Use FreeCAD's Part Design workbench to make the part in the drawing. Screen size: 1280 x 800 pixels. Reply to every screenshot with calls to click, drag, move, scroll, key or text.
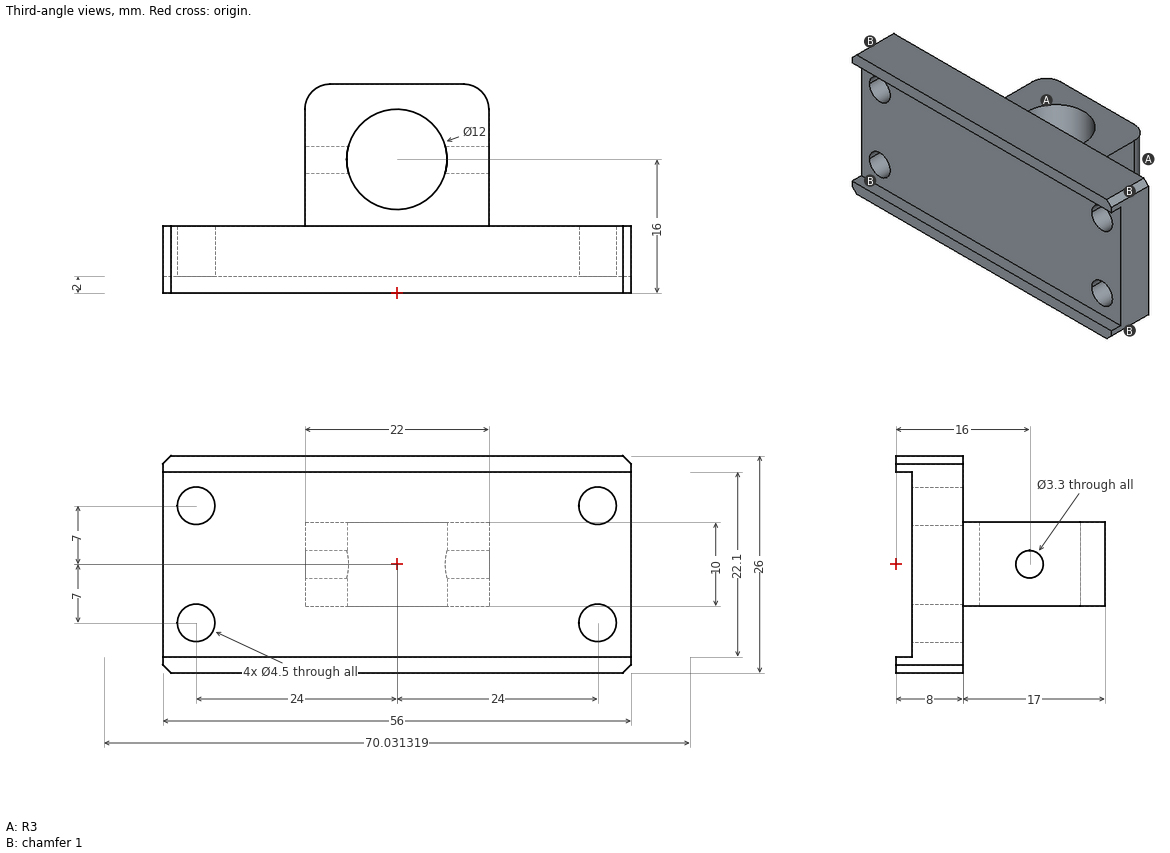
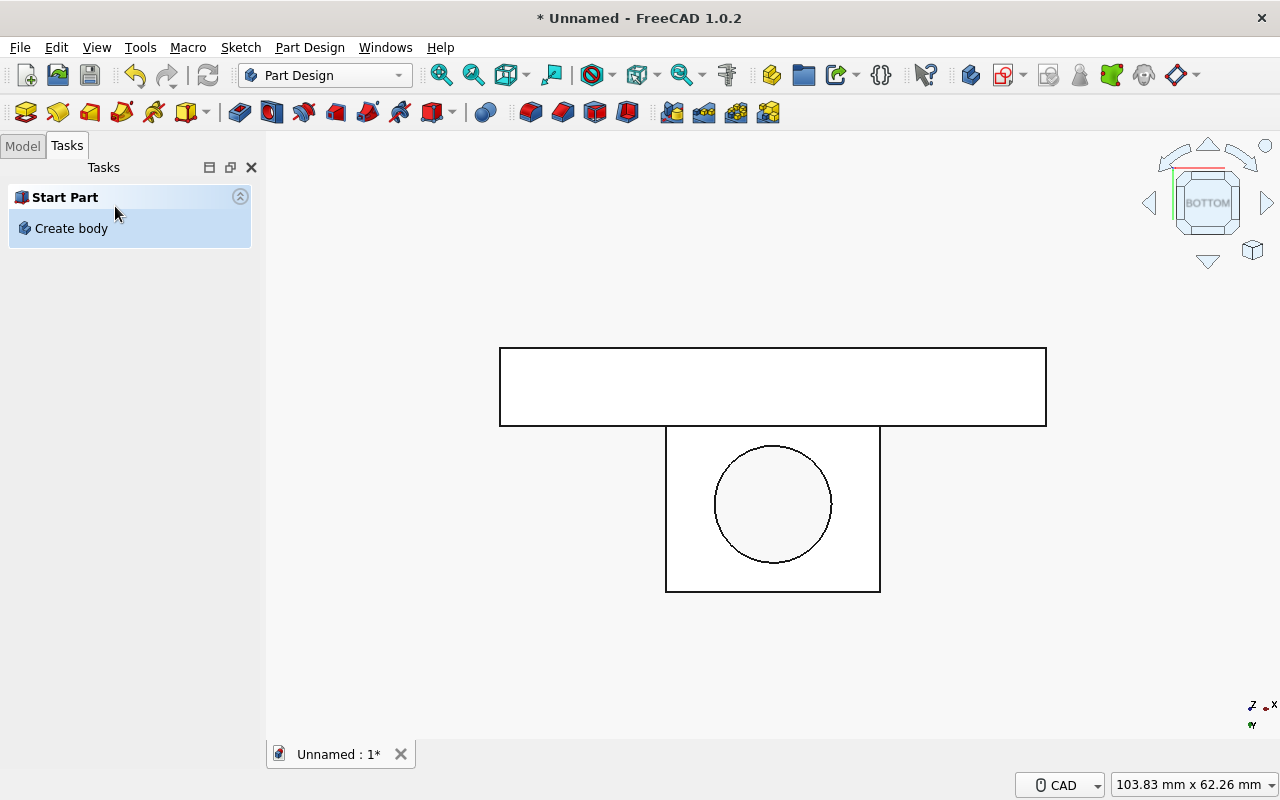
key(4)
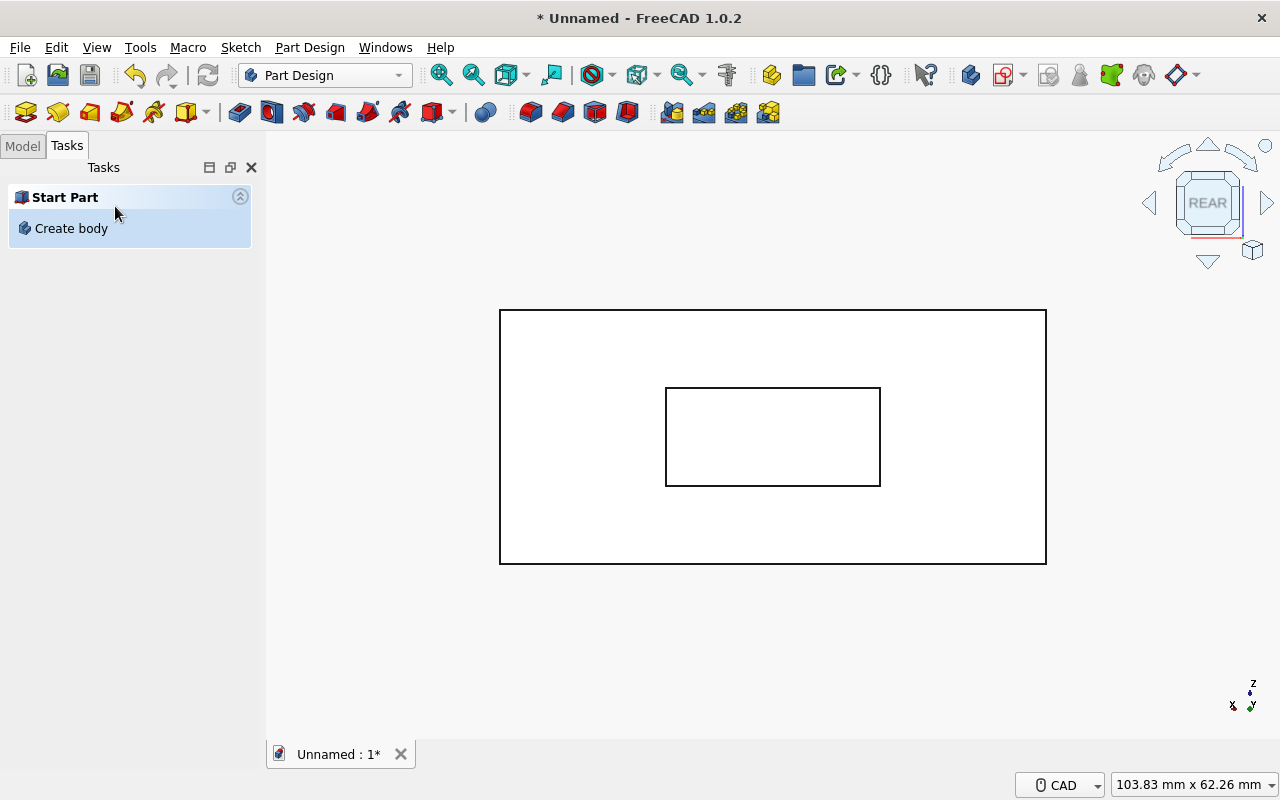
click(617, 508)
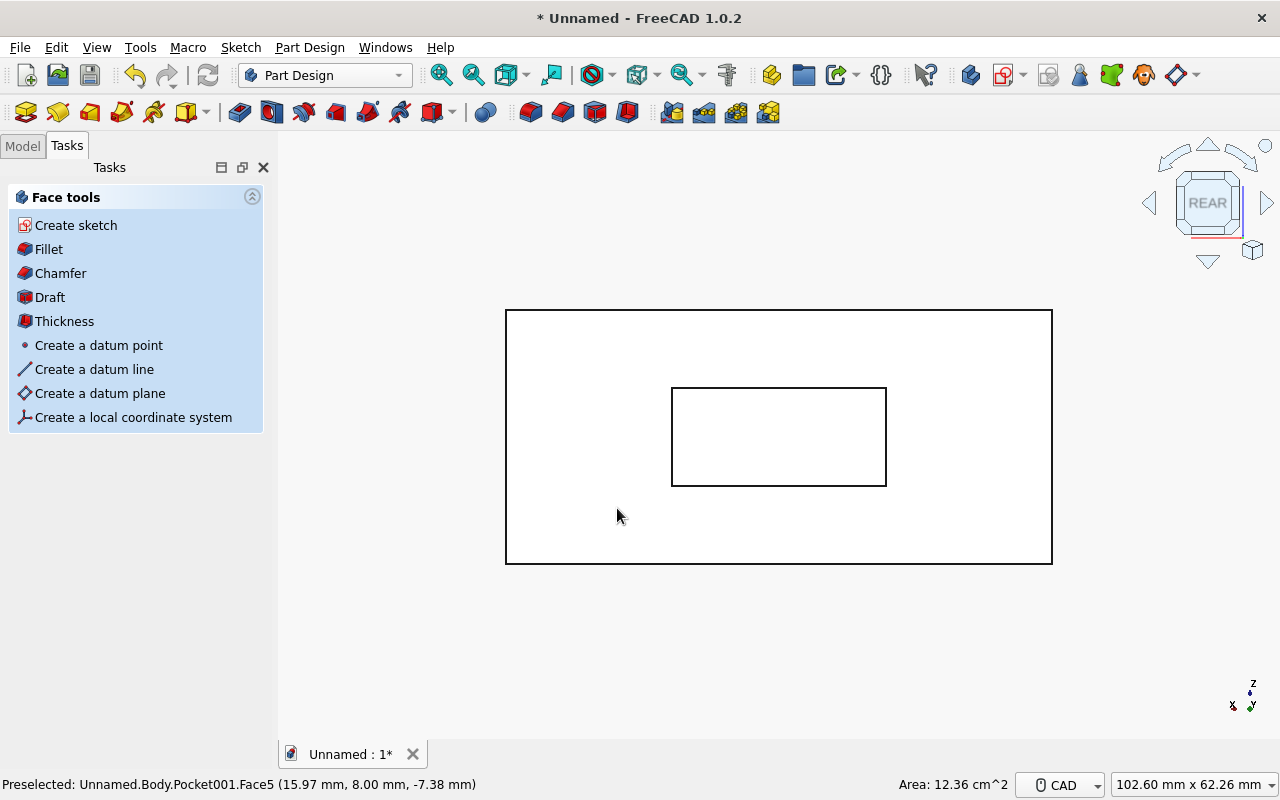
click(1004, 76)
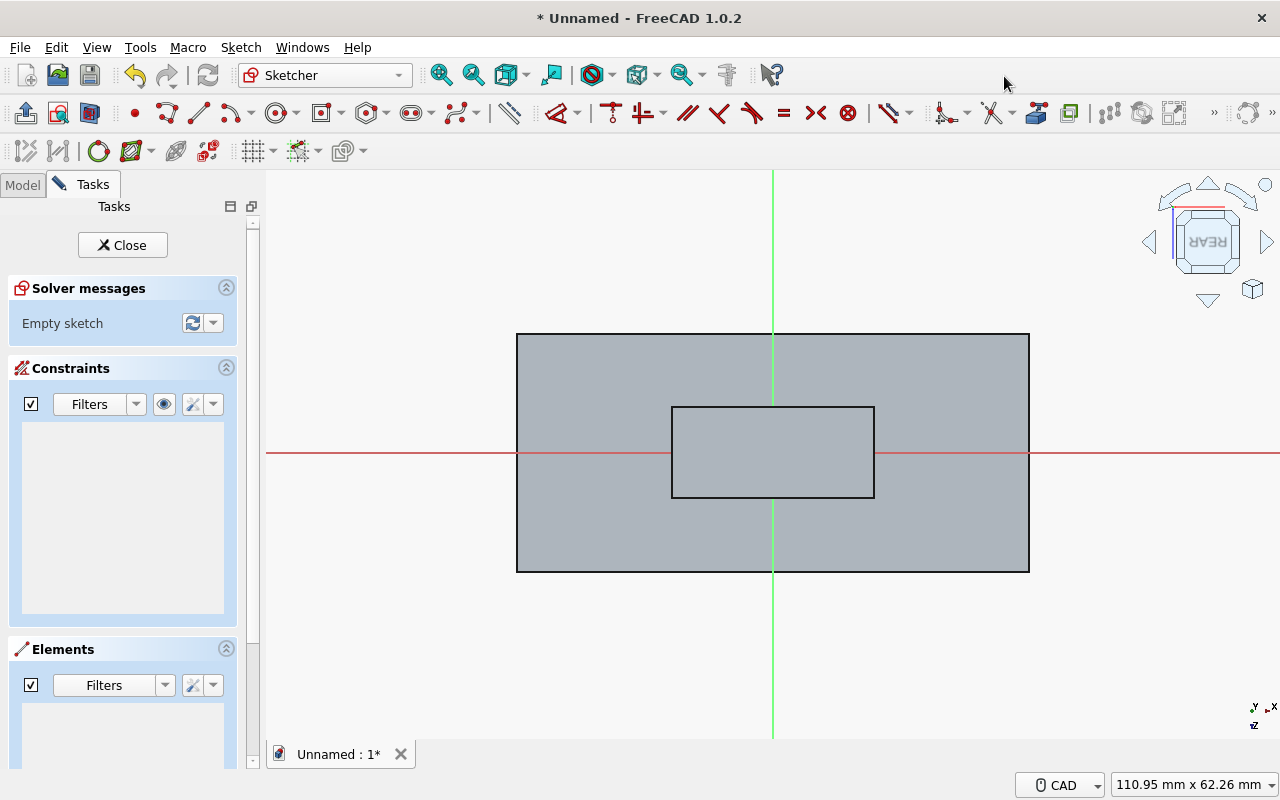
click(276, 114)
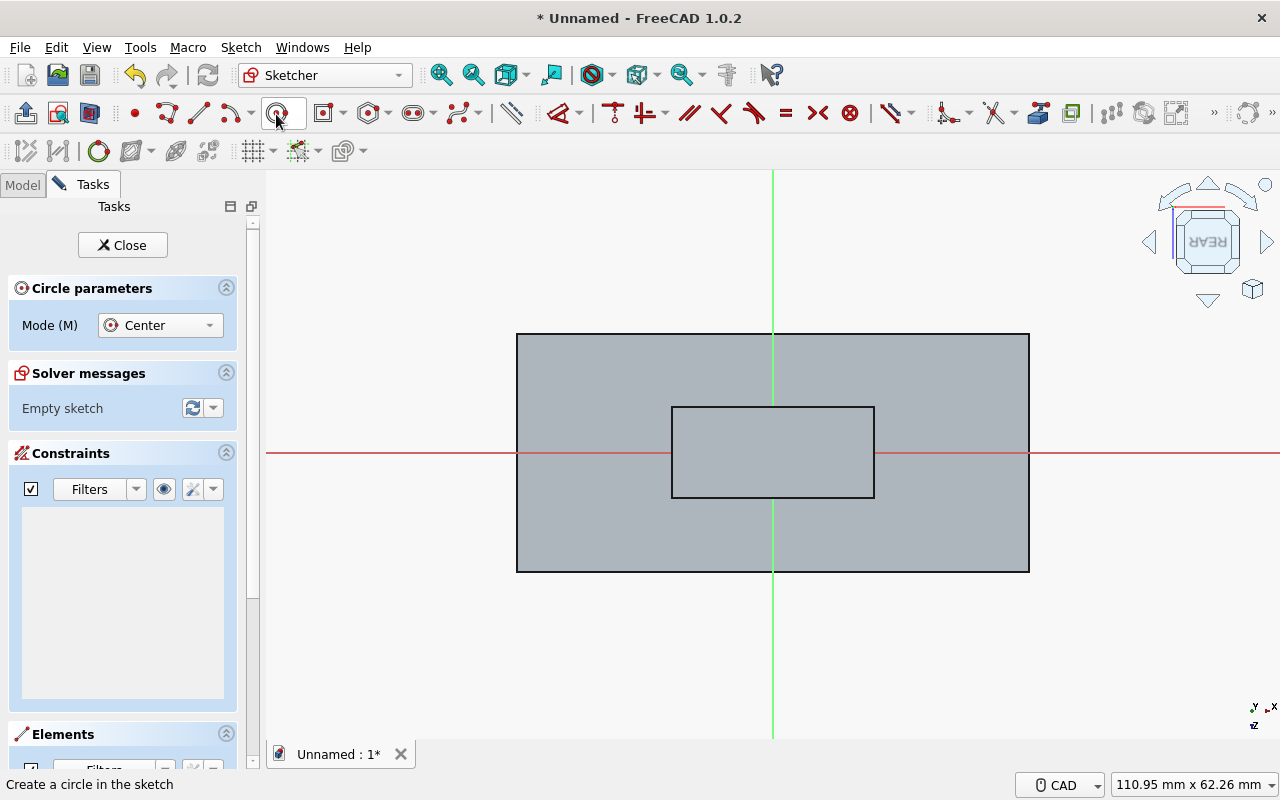
click(554, 389)
move(568, 374)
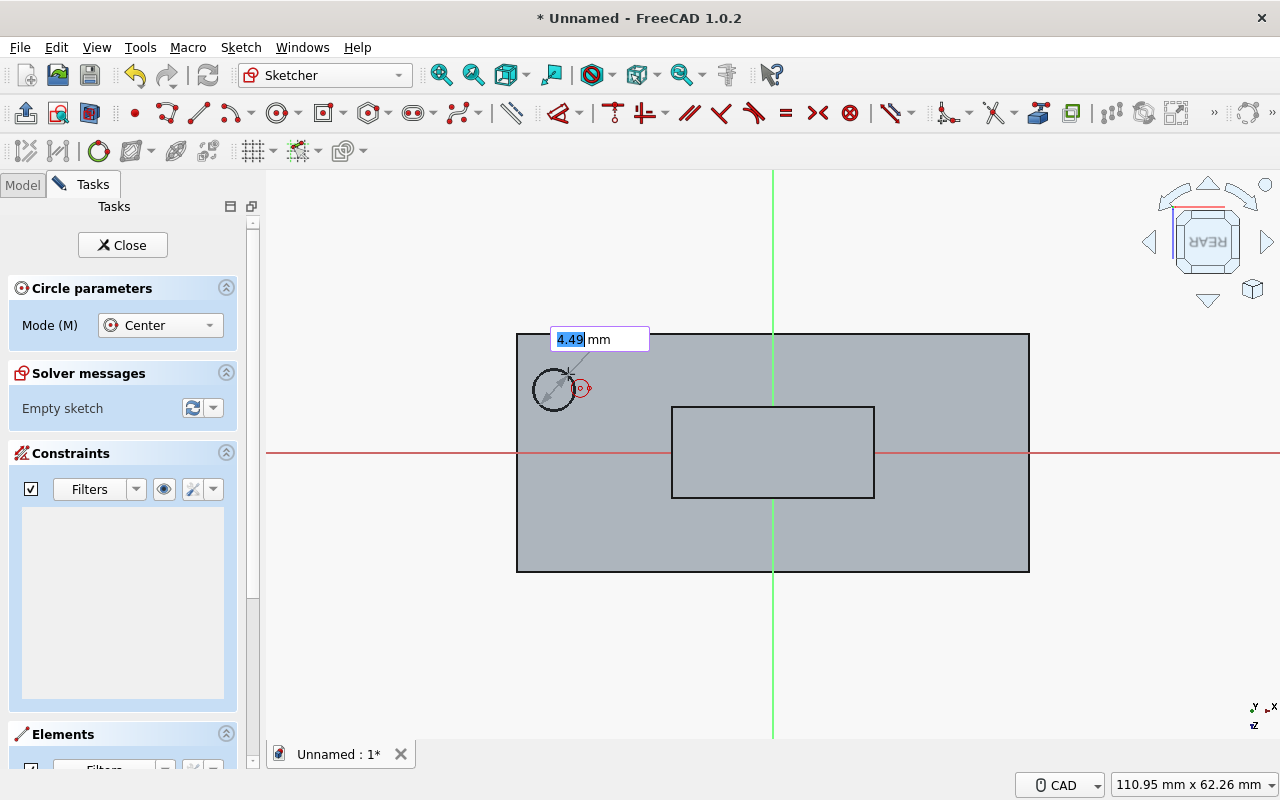
text(4.5)
key(Return)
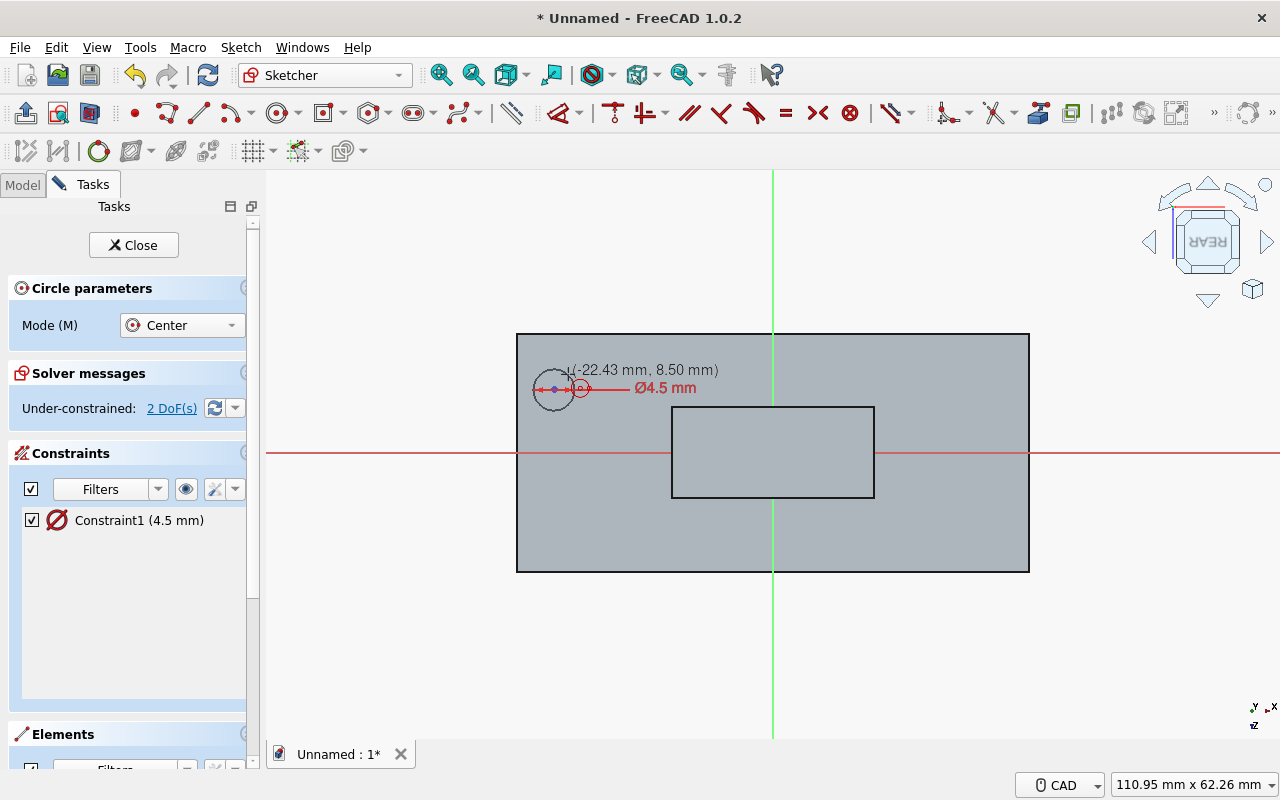
click(554, 517)
move(568, 502)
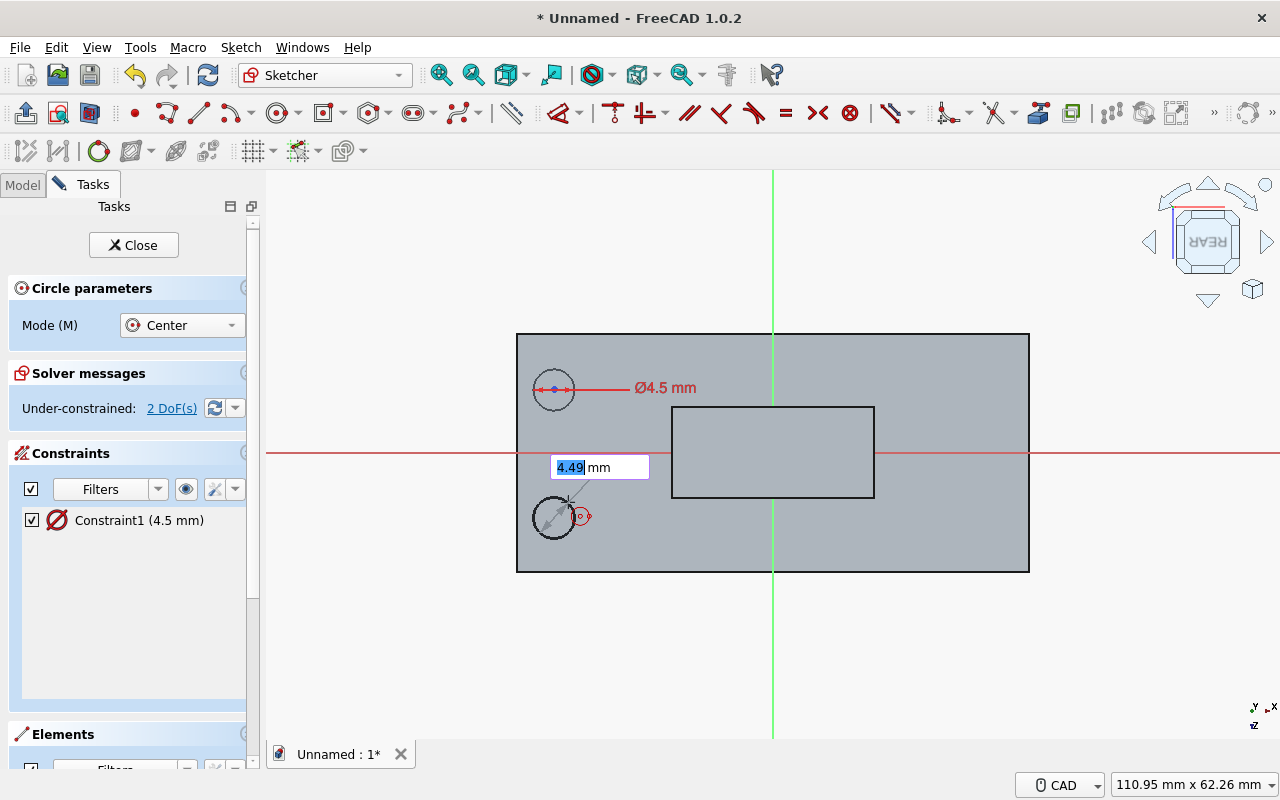
text(4.5)
key(Return)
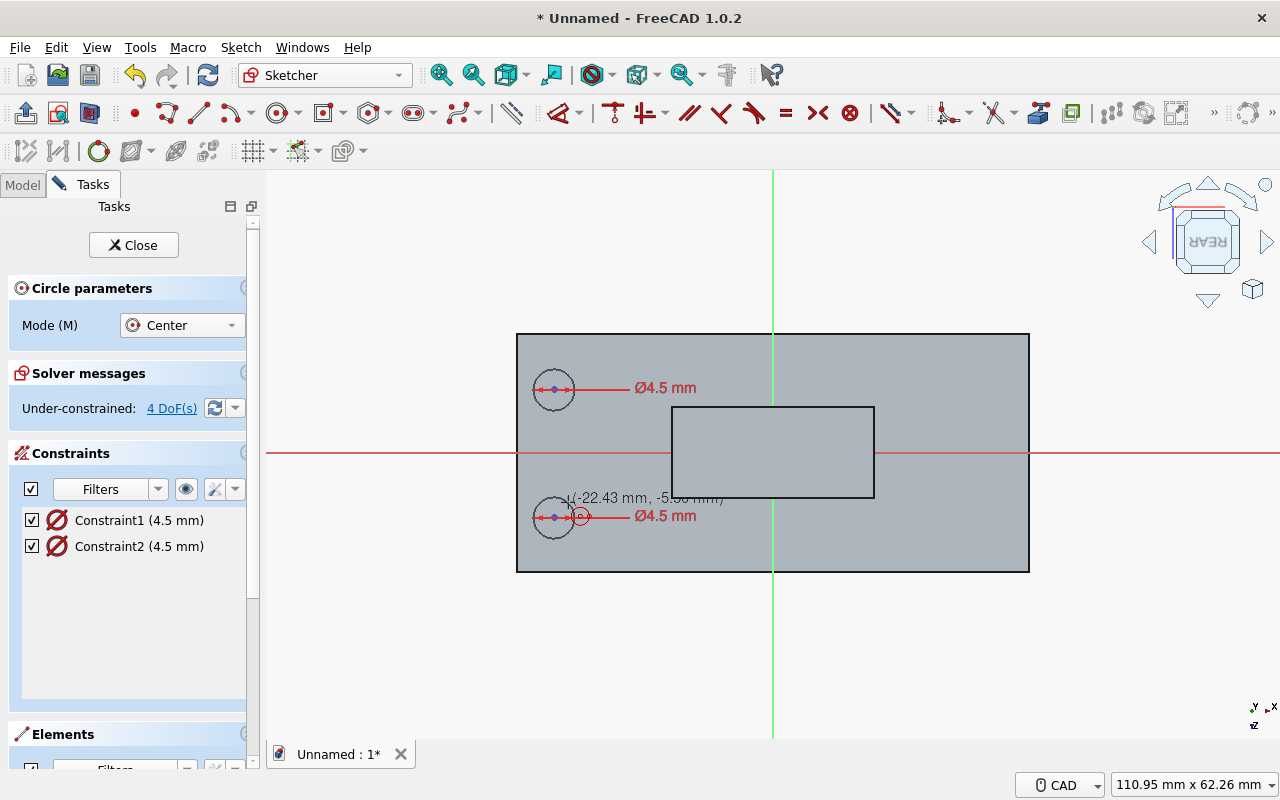
click(992, 389)
move(1007, 374)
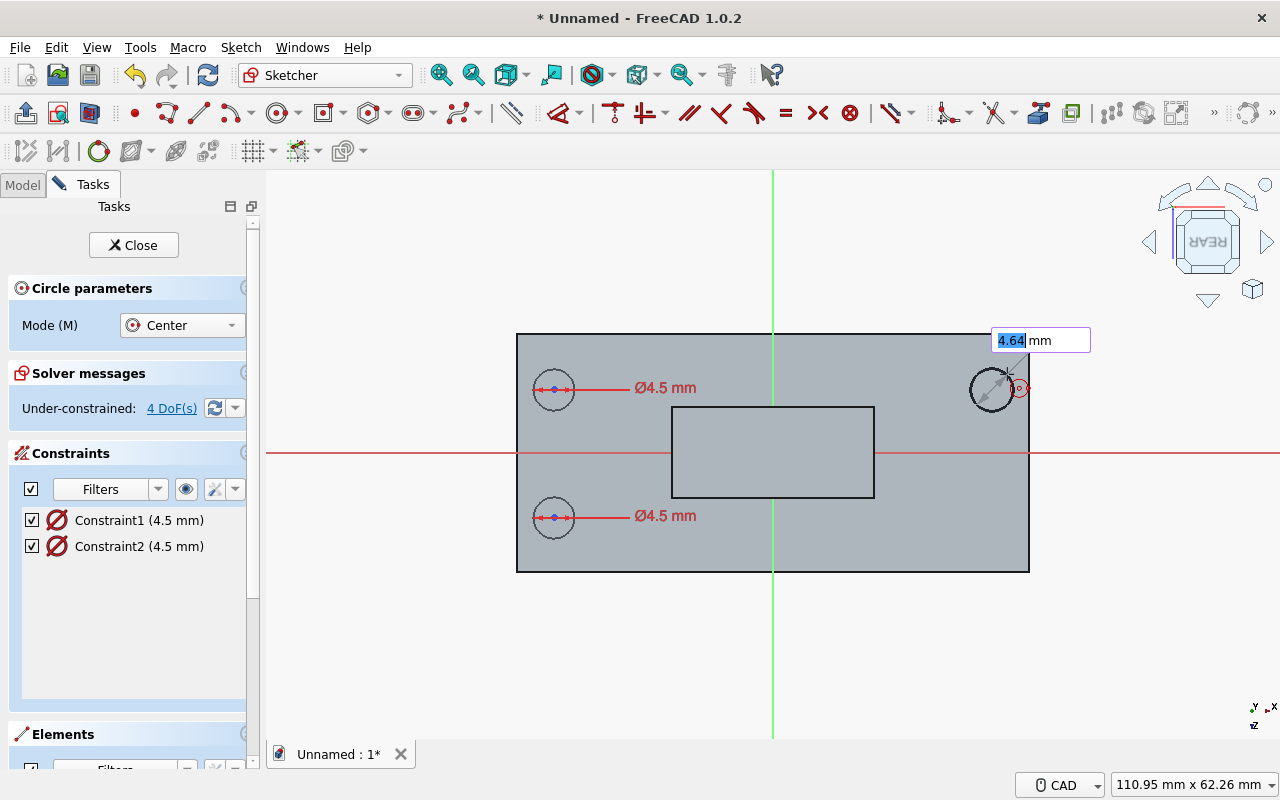
text(4.5)
key(Return)